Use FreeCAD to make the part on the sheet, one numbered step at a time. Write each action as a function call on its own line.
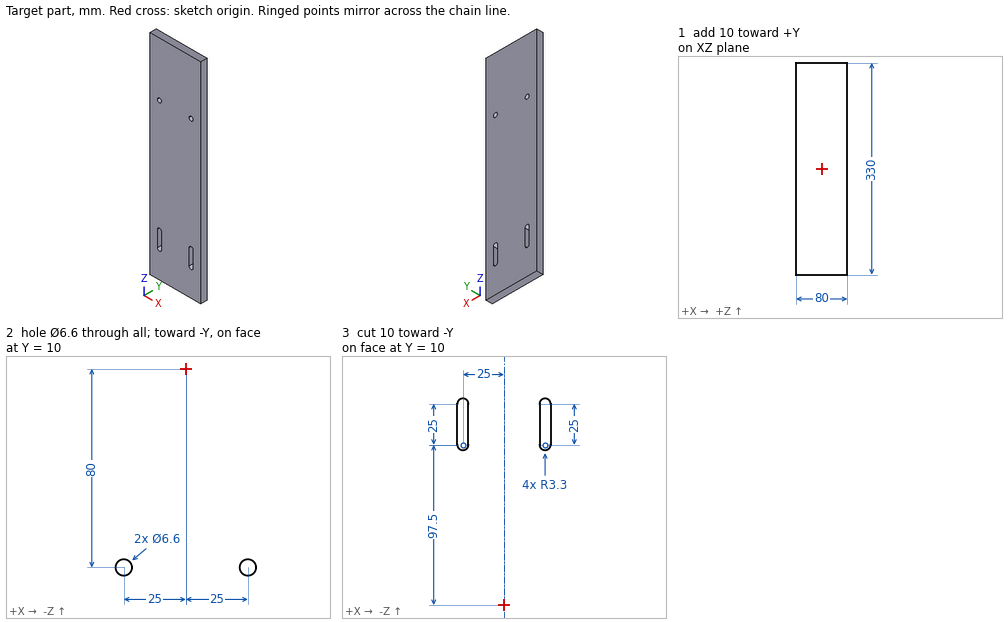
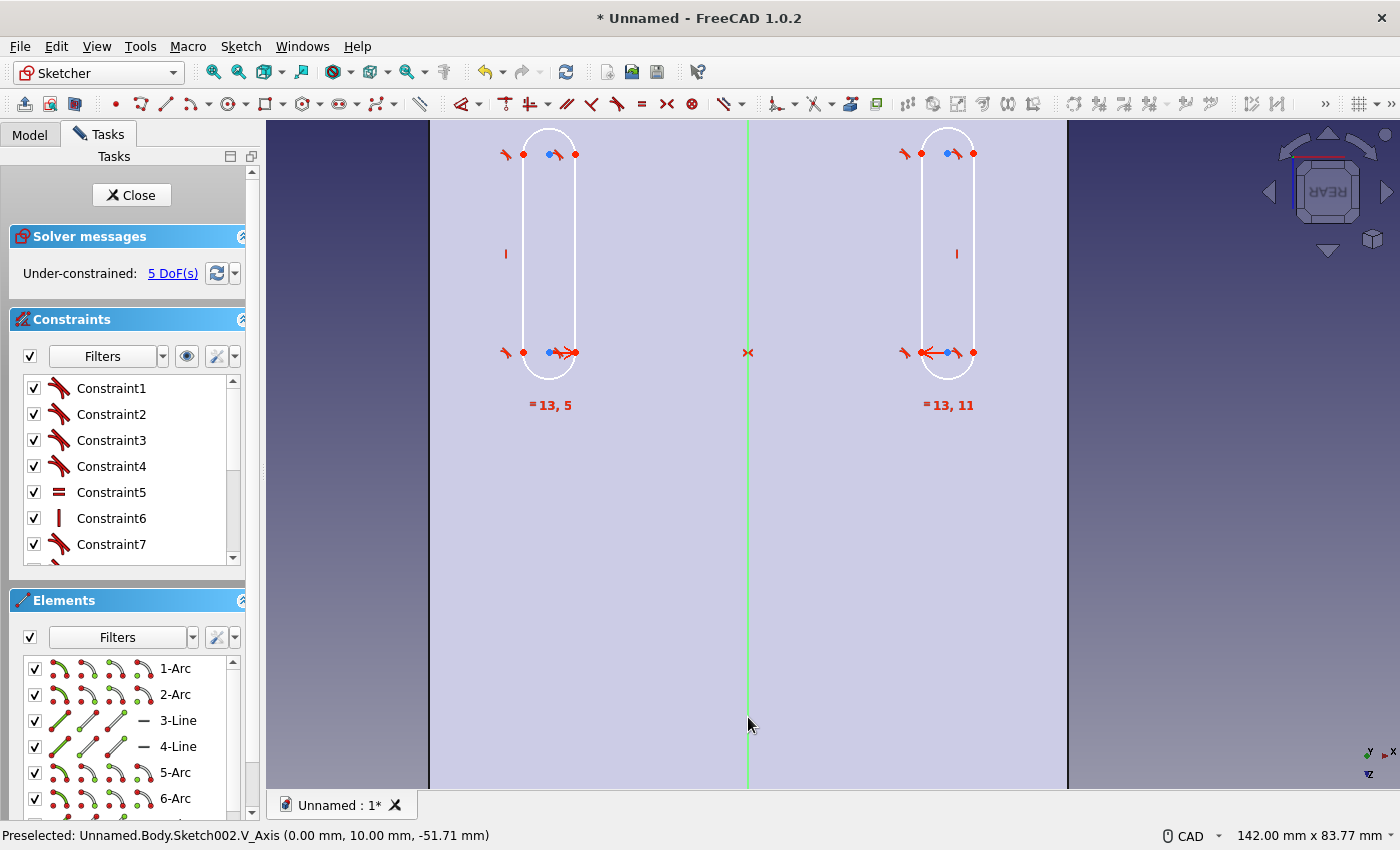
scroll(534, 374, up, 3)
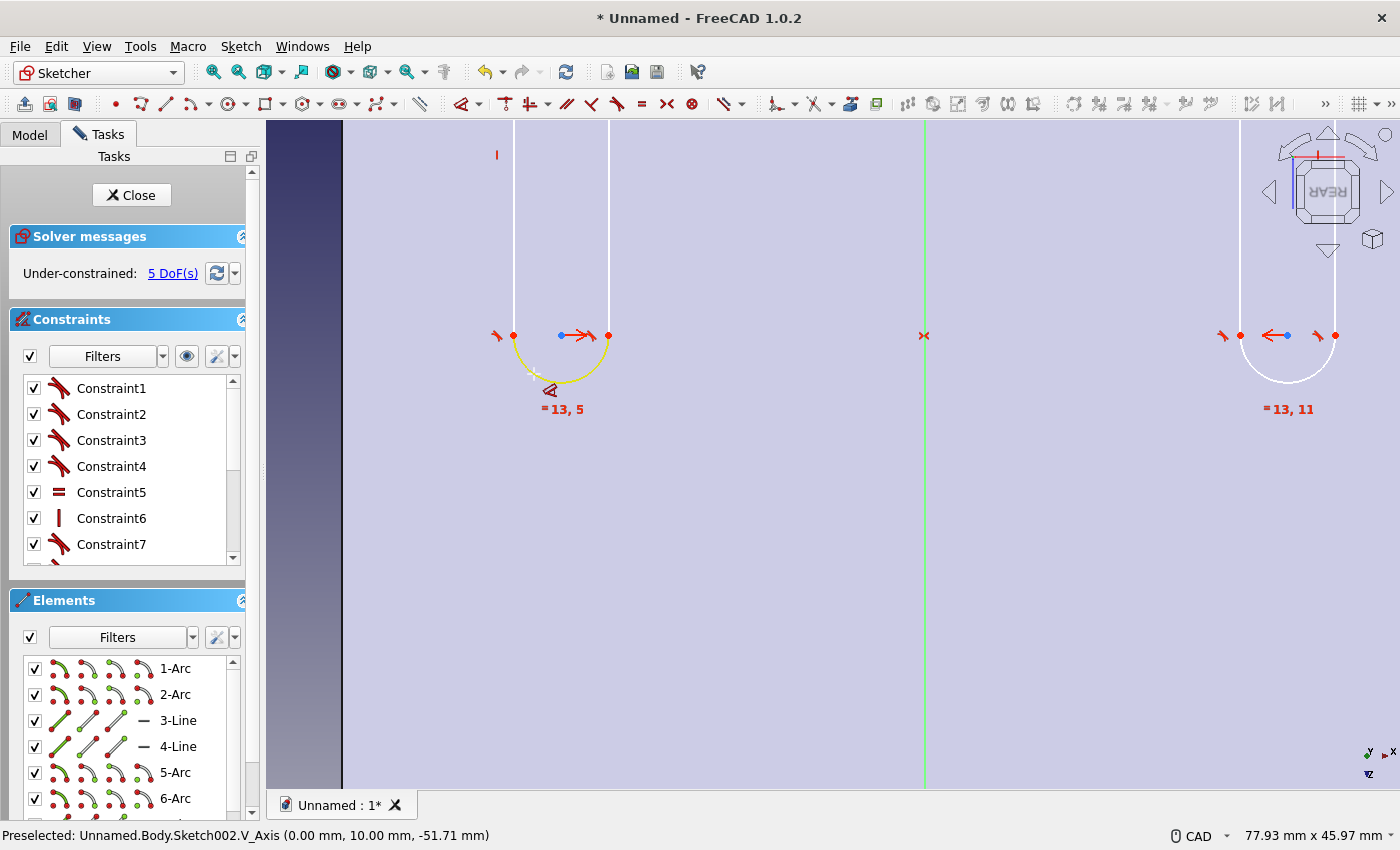
click(533, 374)
click(514, 400)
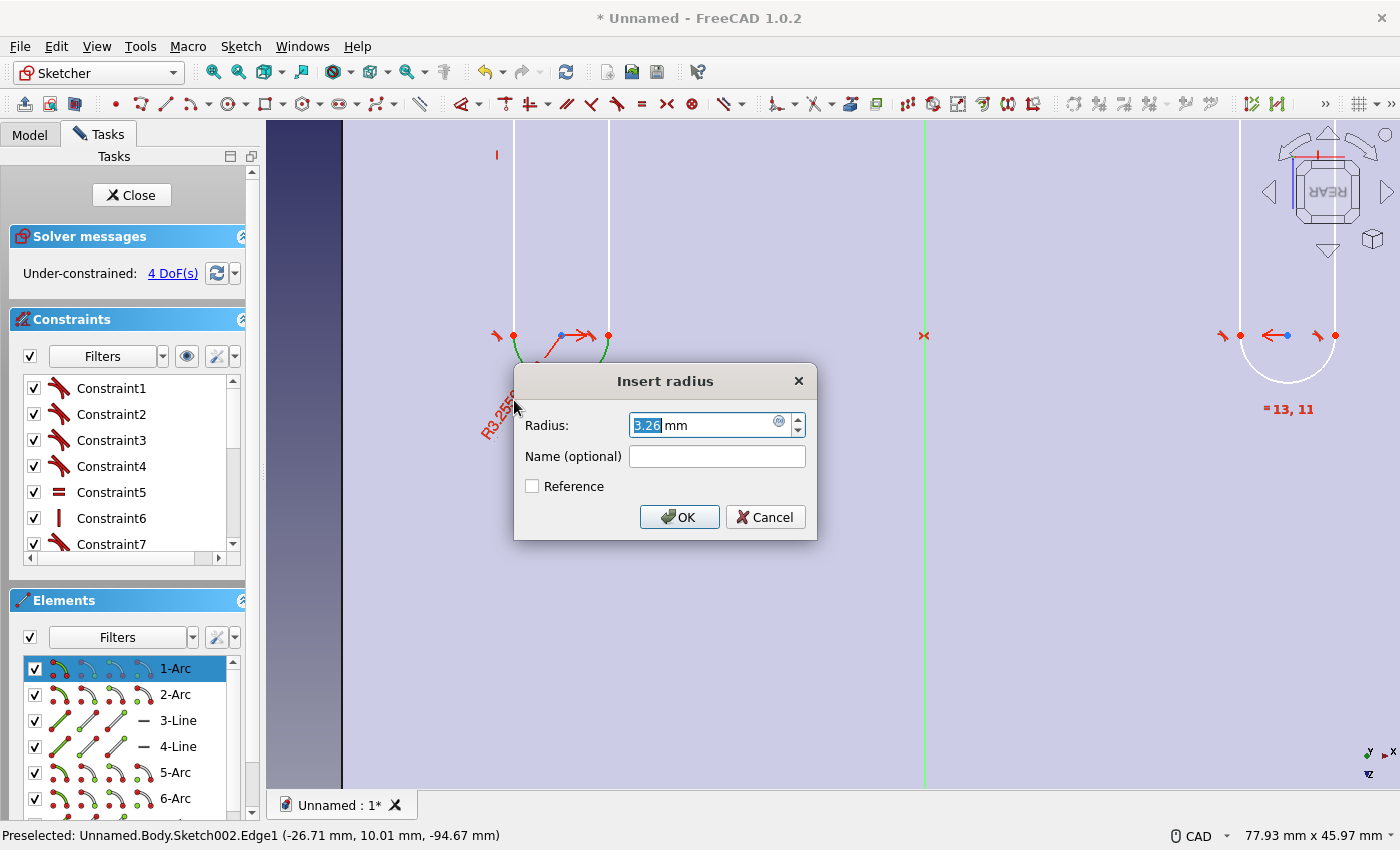
text(3.3)
key(Return)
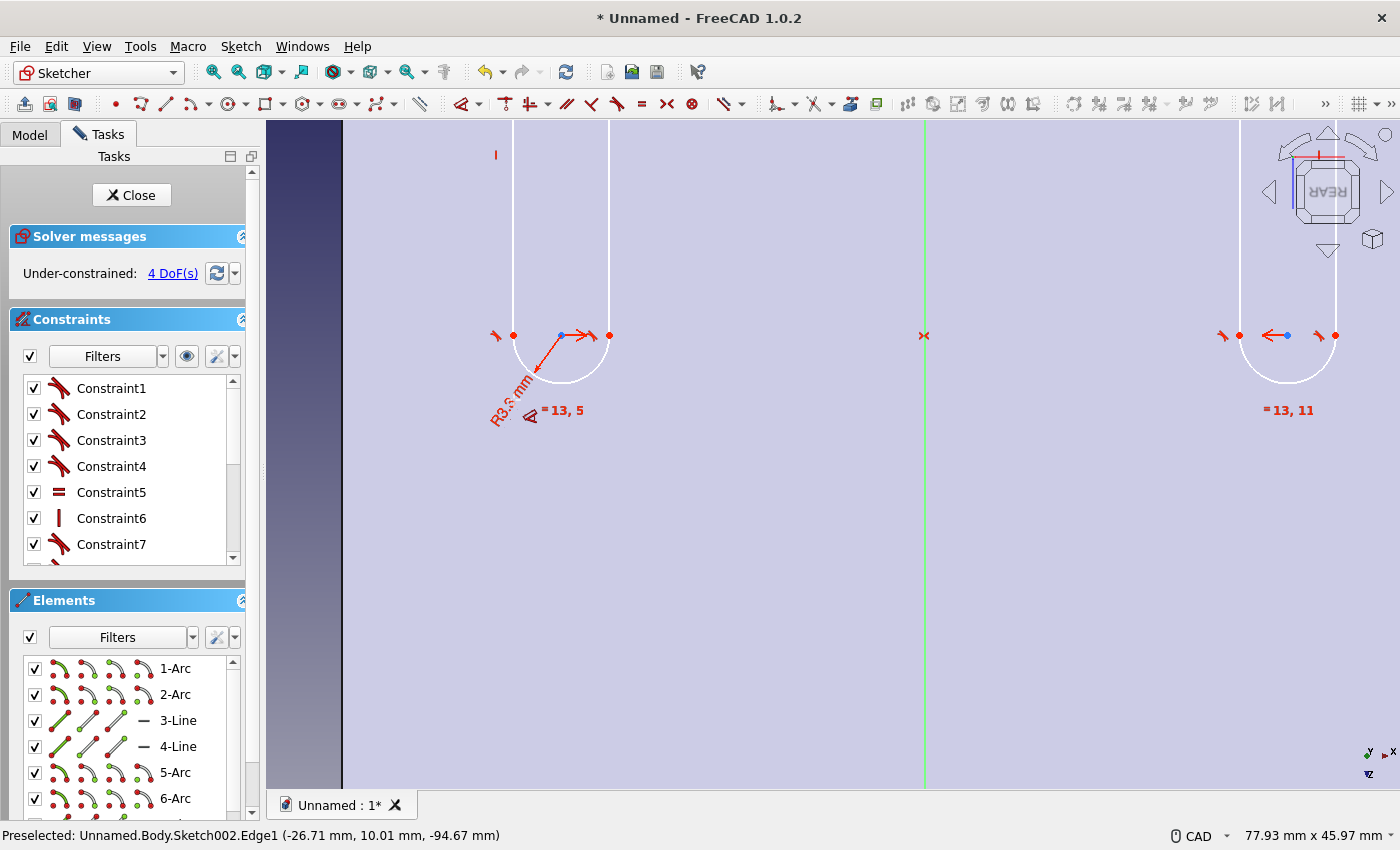
scroll(712, 329, down, 7)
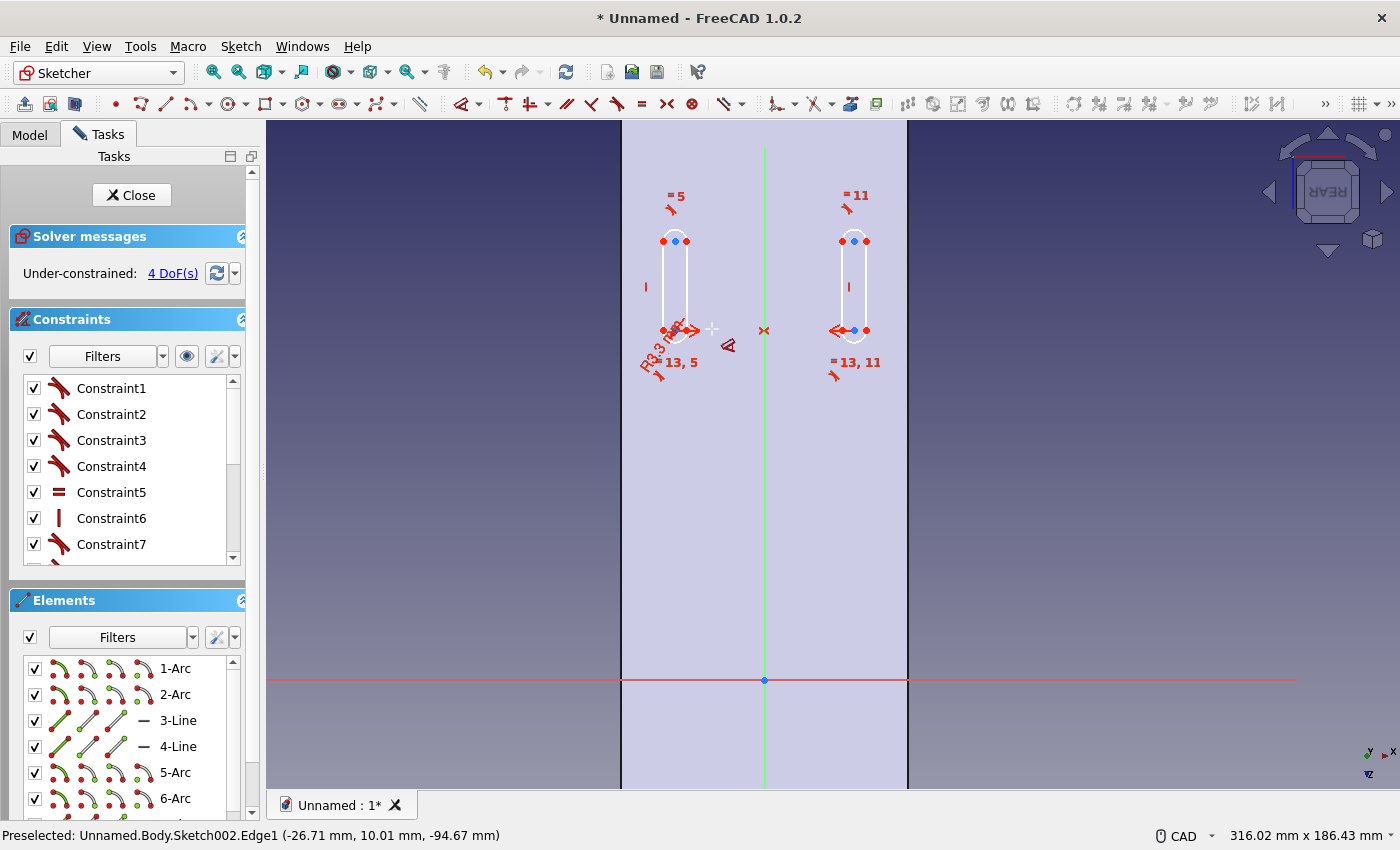
click(663, 304)
click(629, 286)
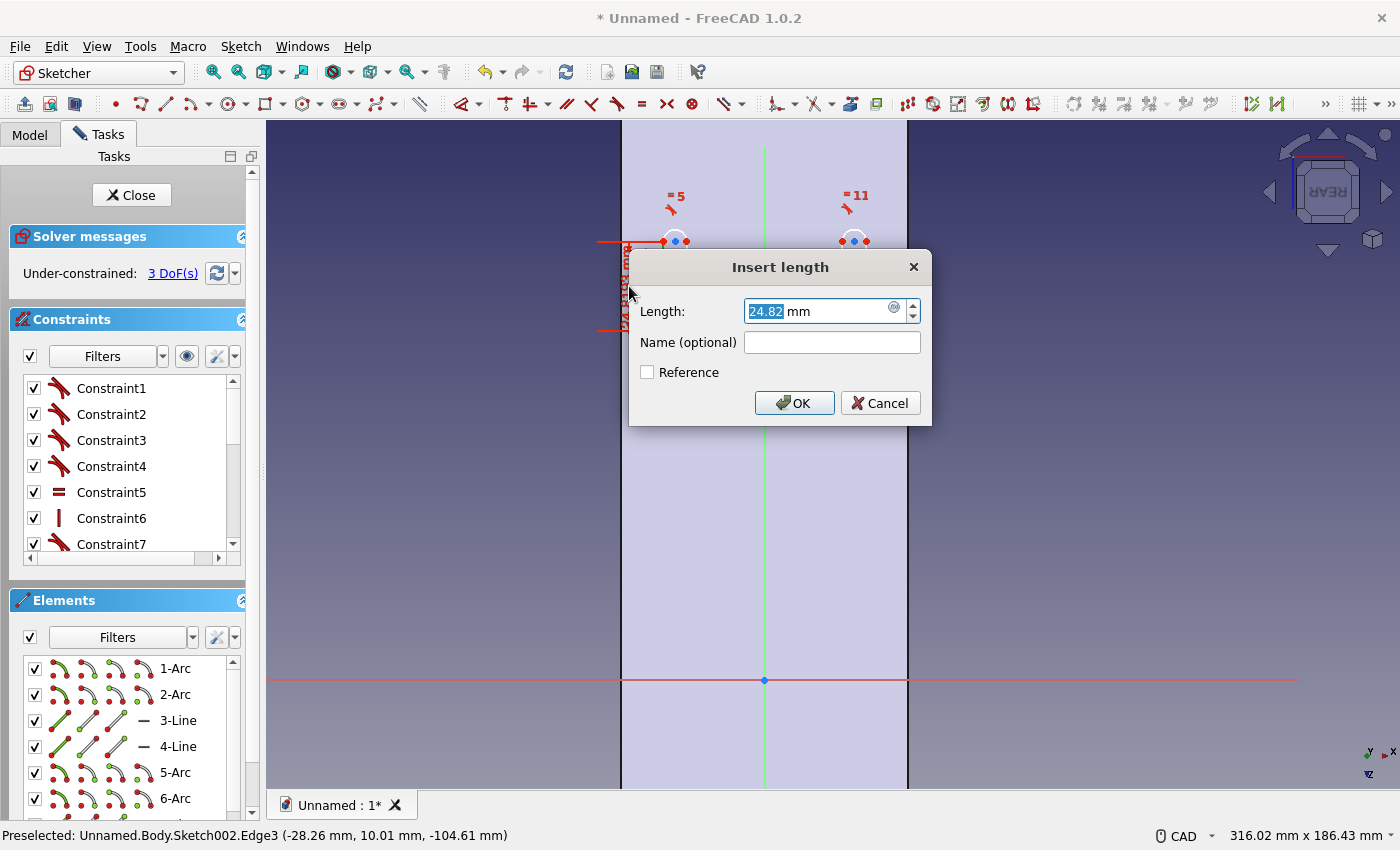
text(25)
key(Return)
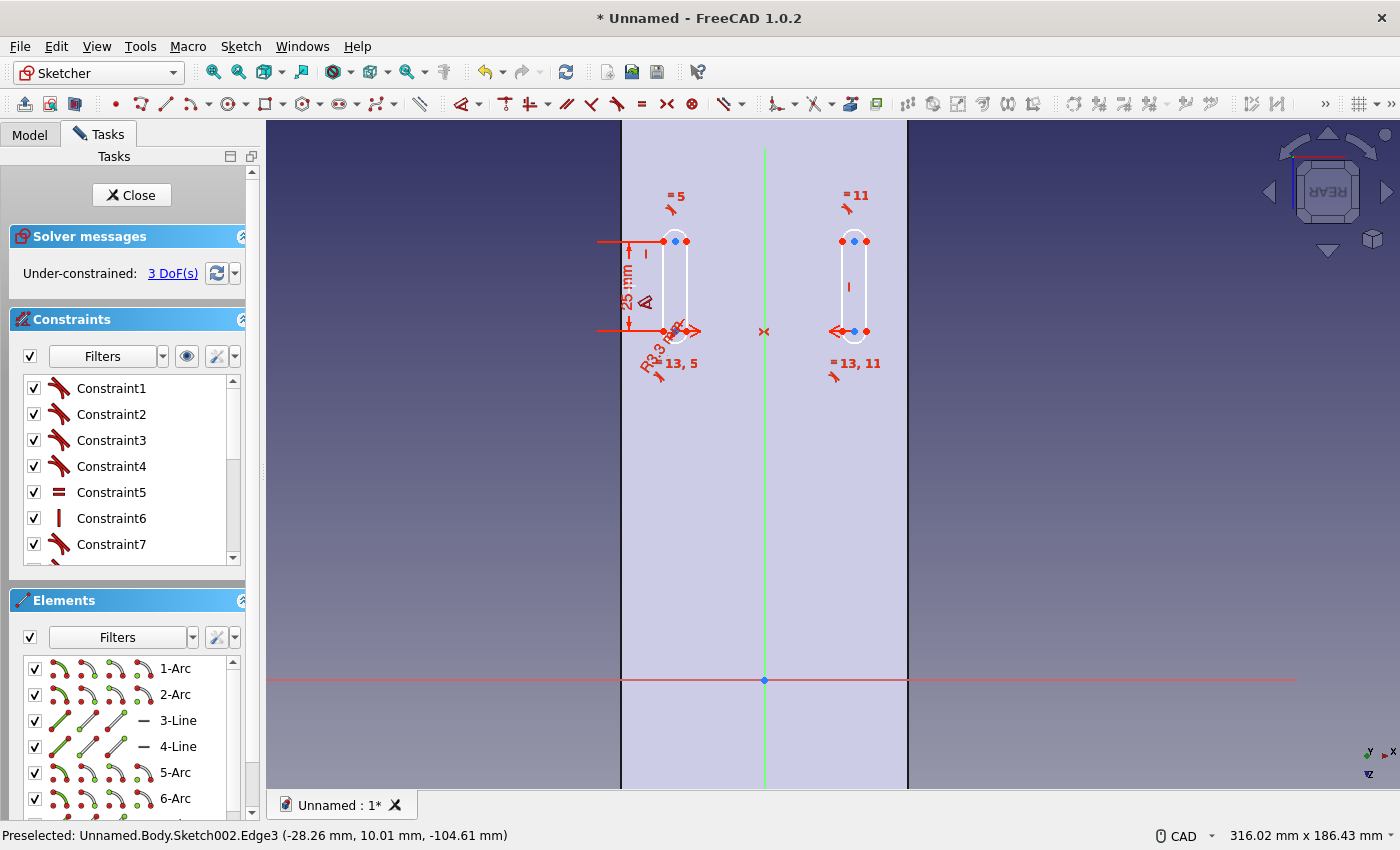
click(842, 304)
click(808, 286)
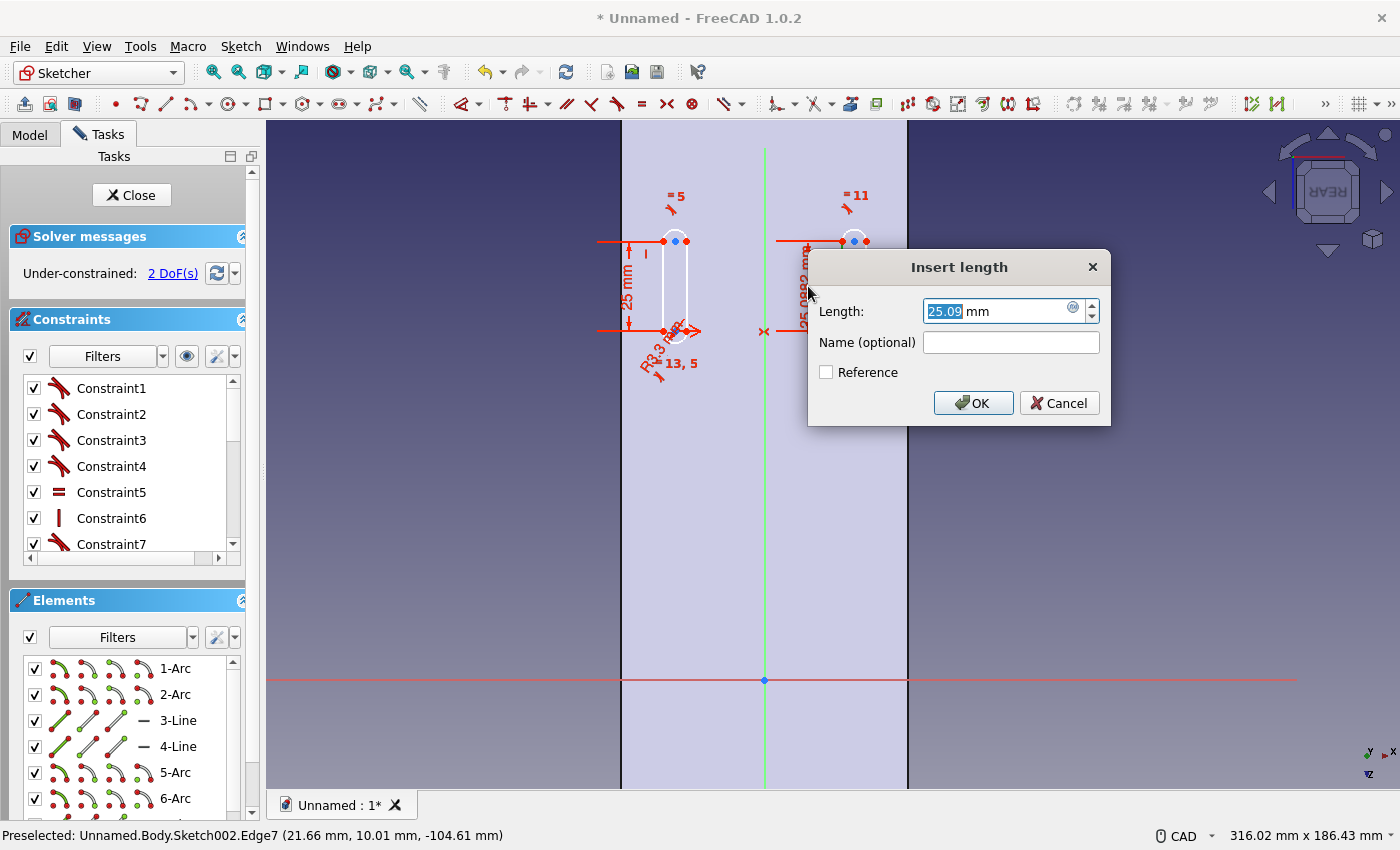
text(25)
key(Return)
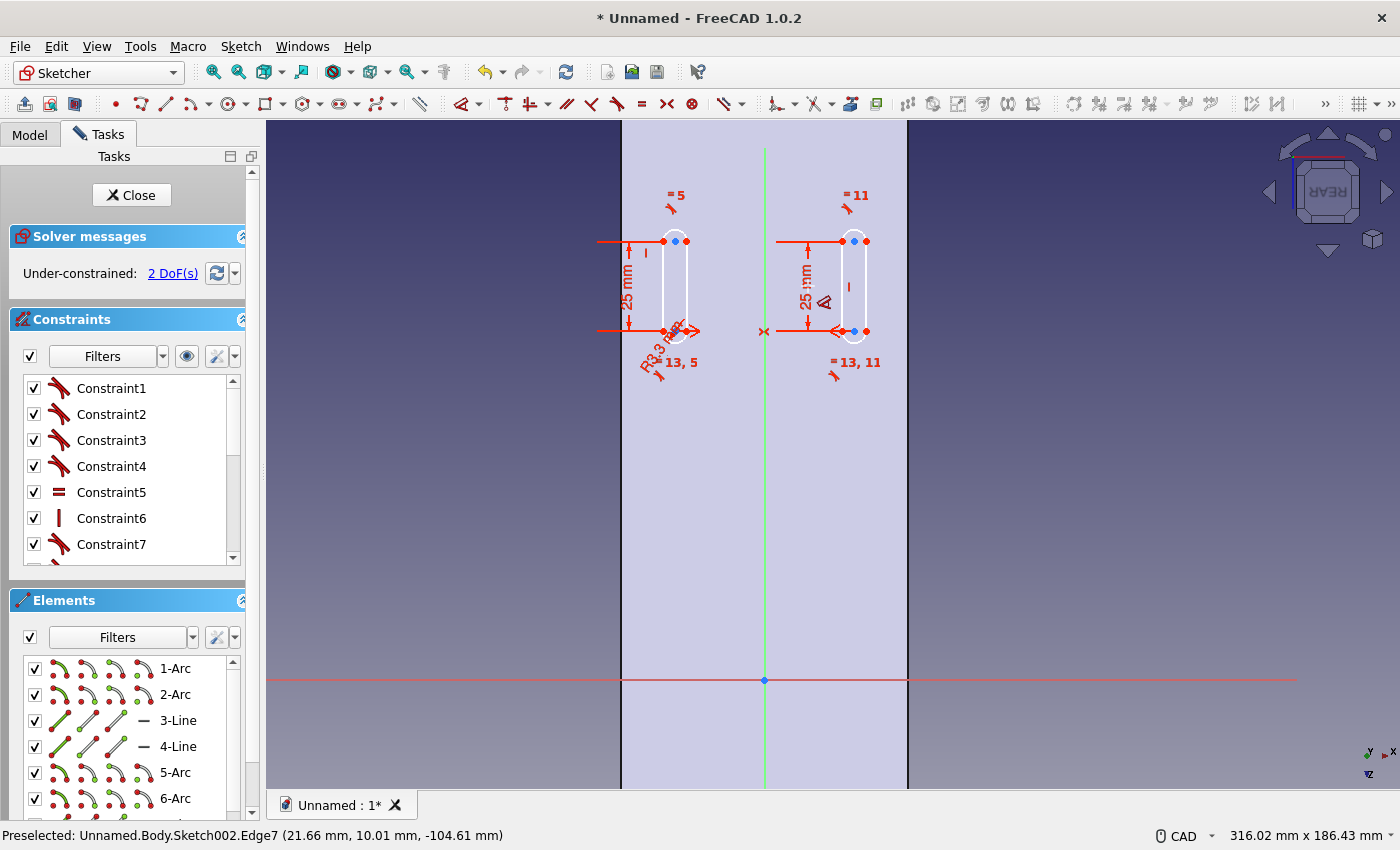
click(675, 331)
click(720, 714)